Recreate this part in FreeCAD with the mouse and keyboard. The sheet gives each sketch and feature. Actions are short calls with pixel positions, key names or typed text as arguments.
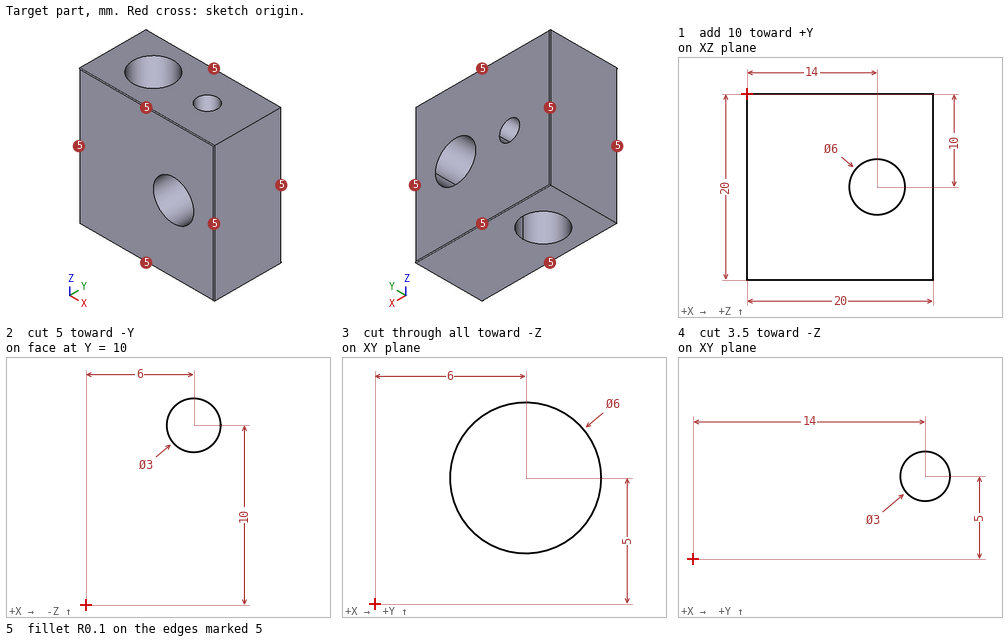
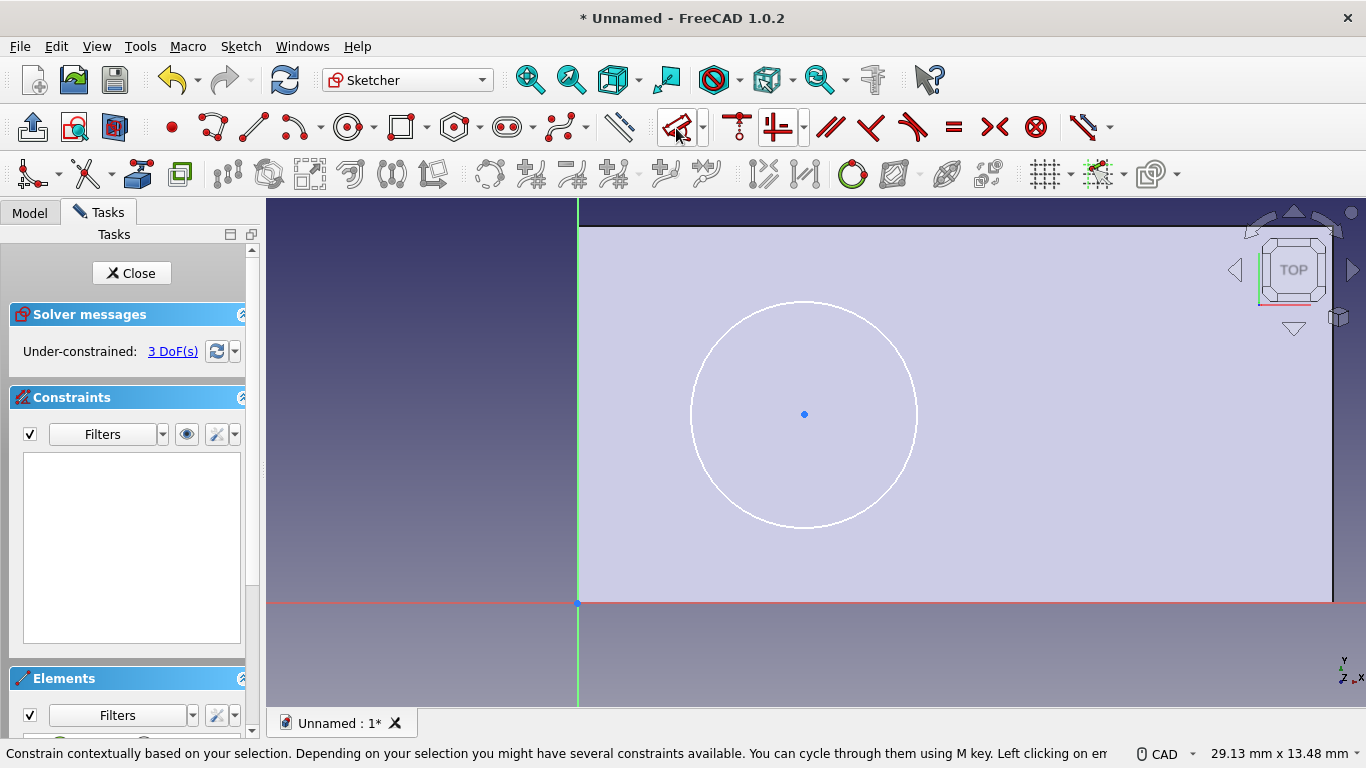
click(884, 335)
click(907, 312)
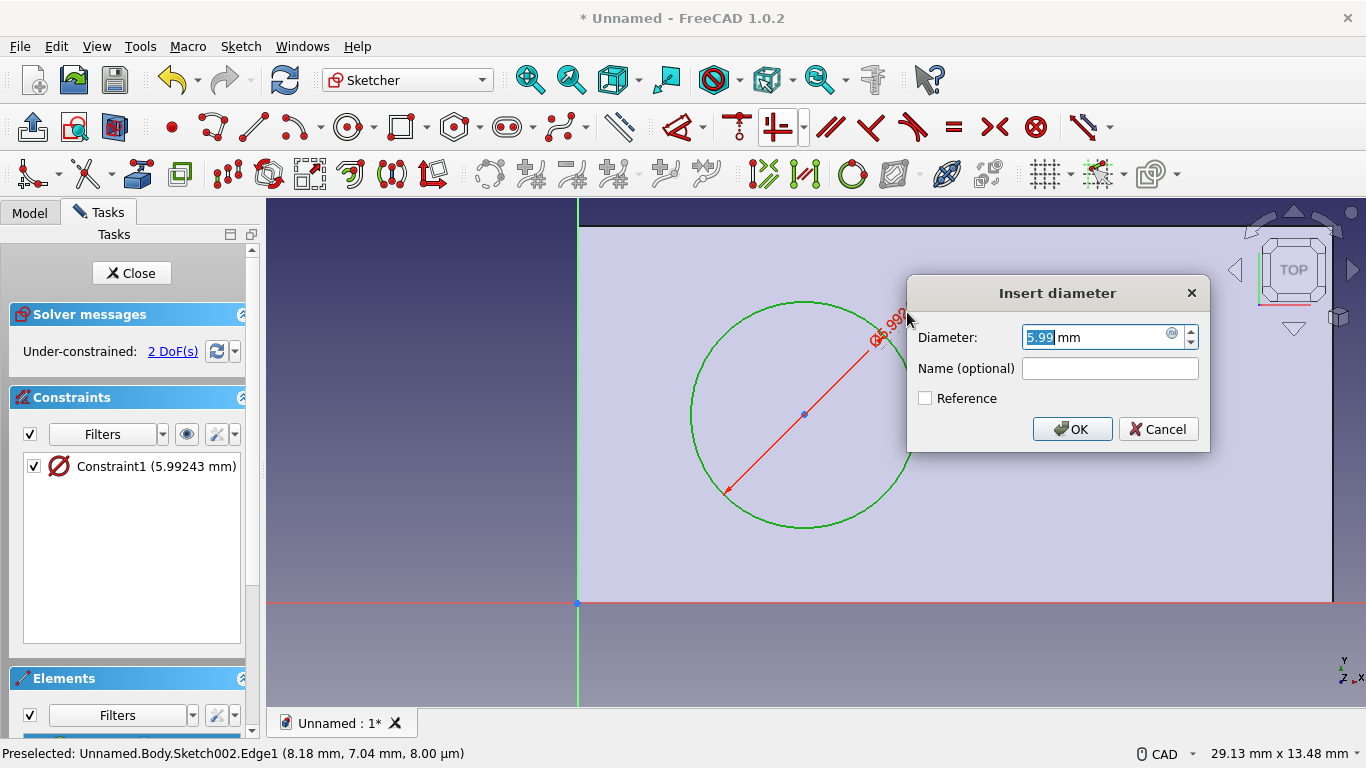
text(6)
key(Return)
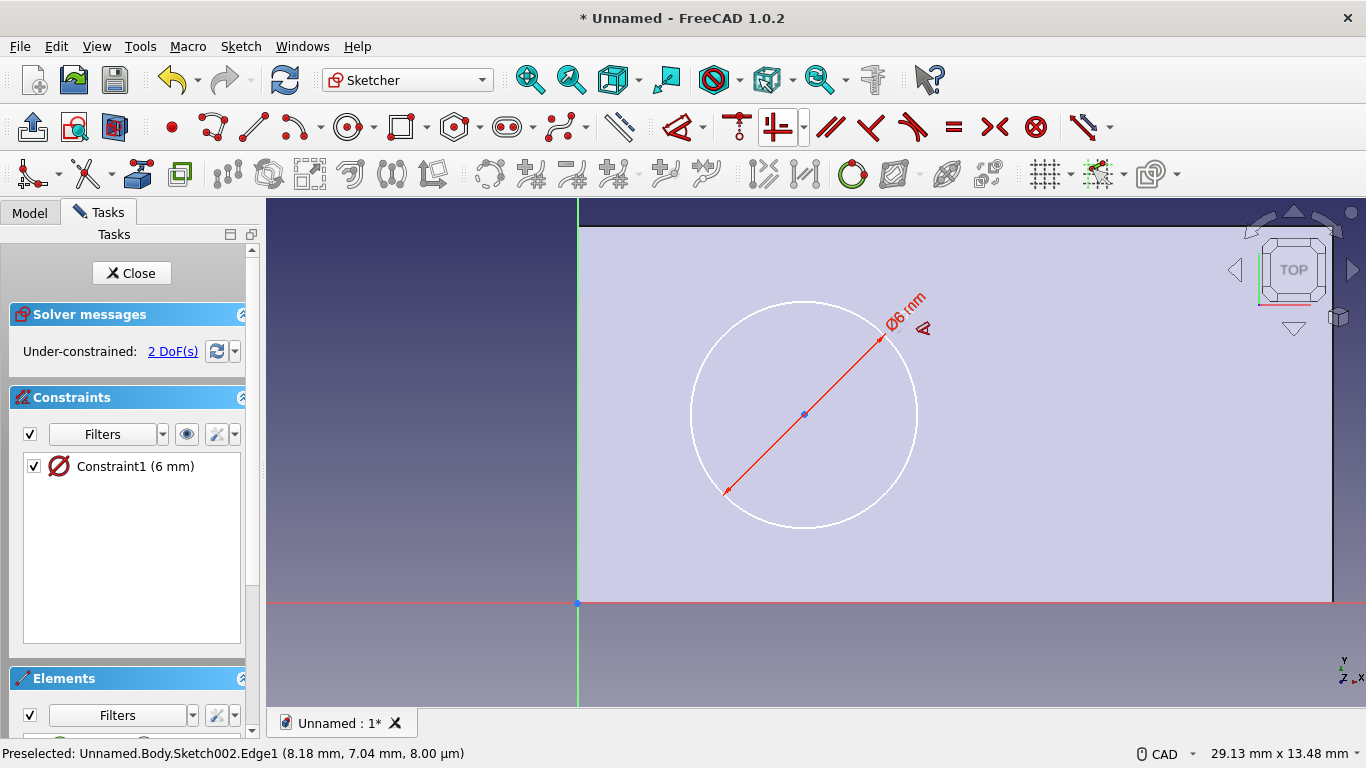
click(804, 415)
click(691, 637)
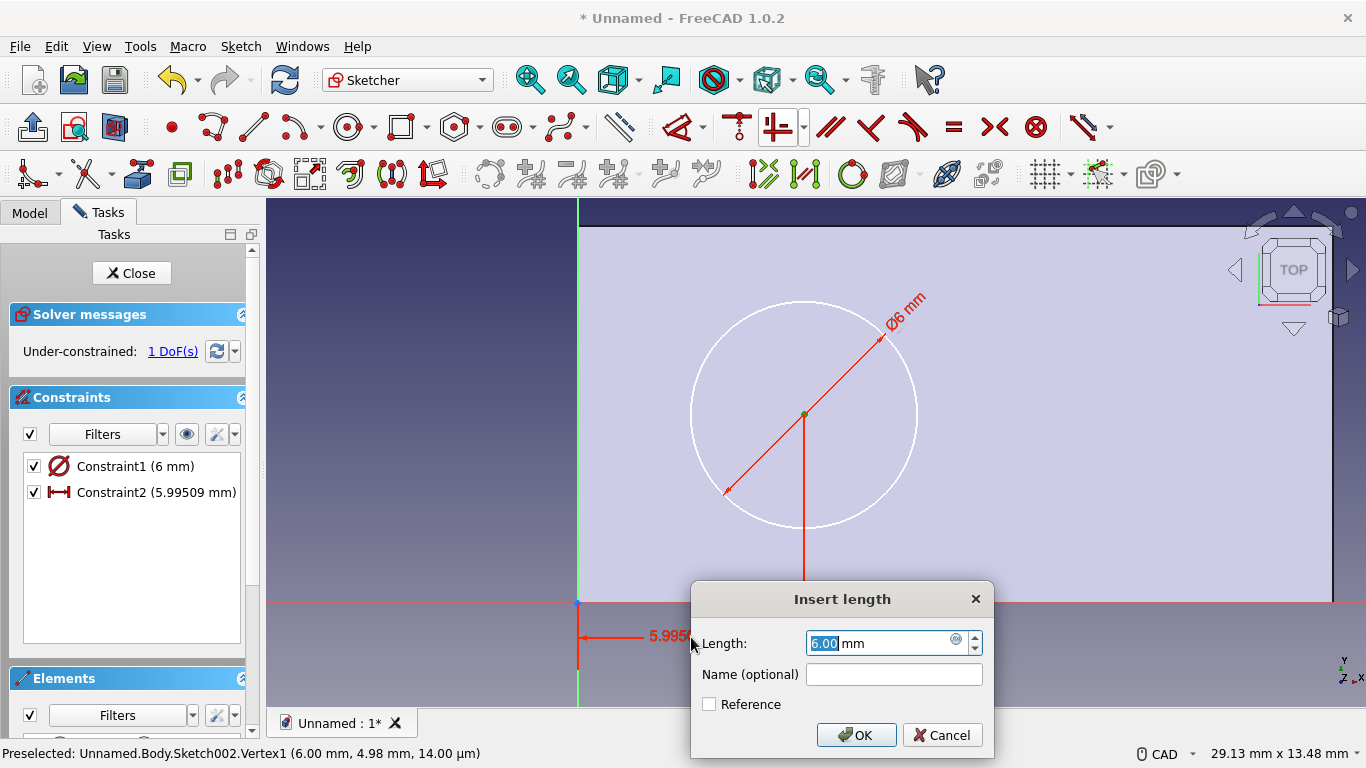
text(6)
key(Return)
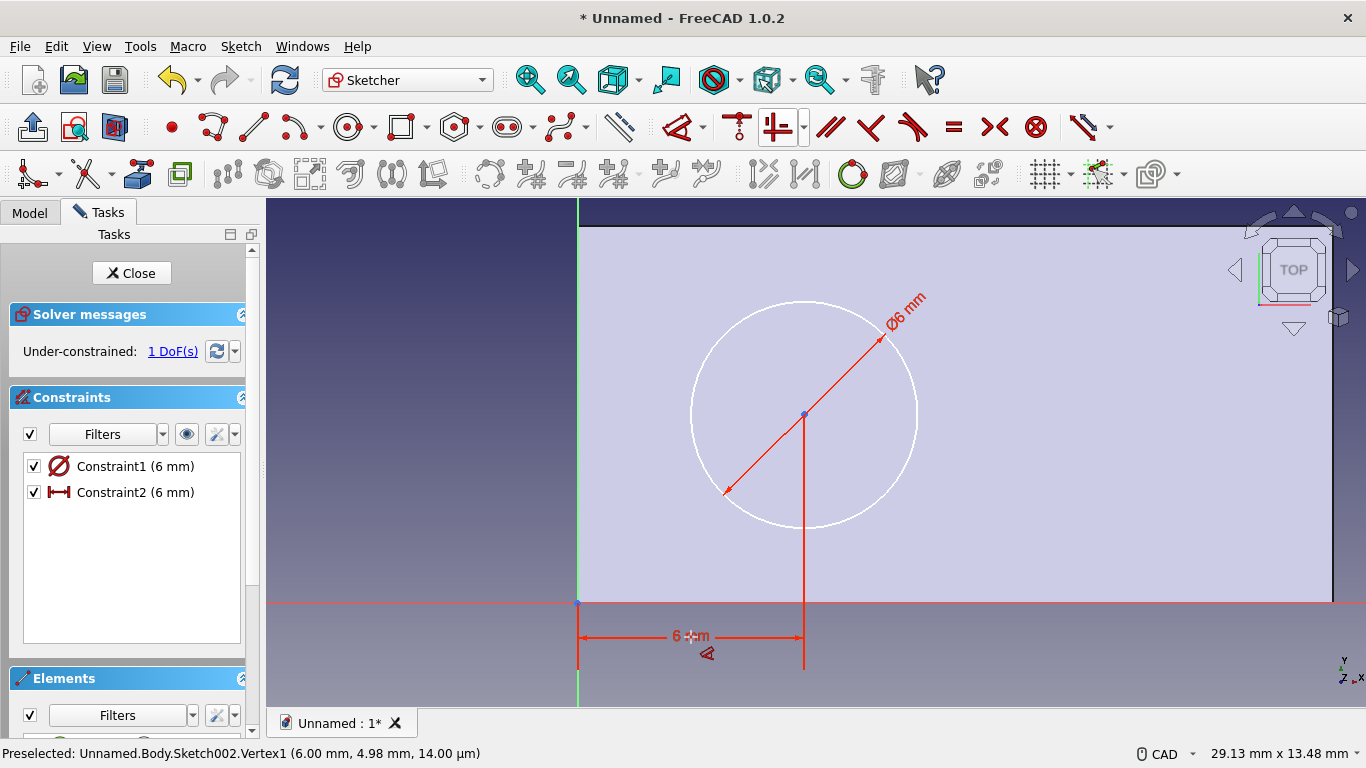
click(804, 415)
click(544, 509)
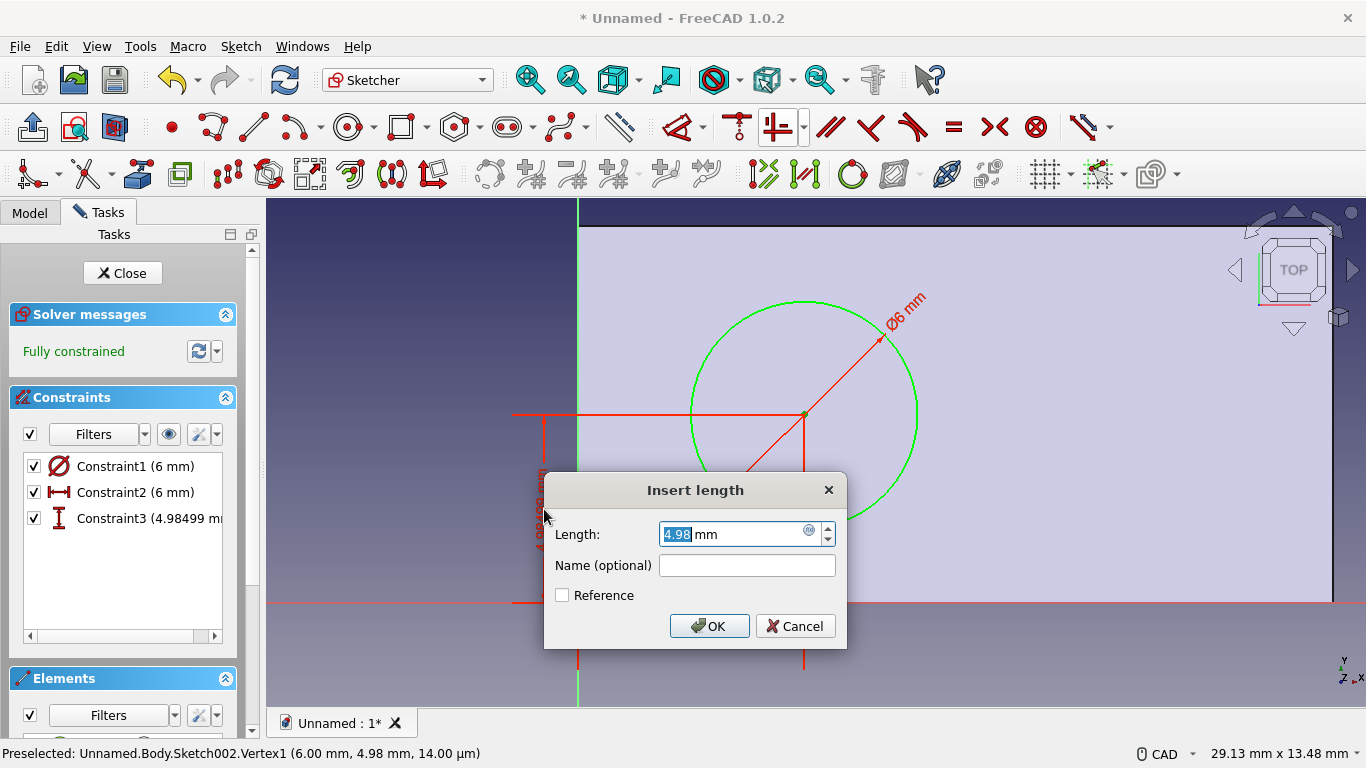
text(5)
key(Return)
key(Escape)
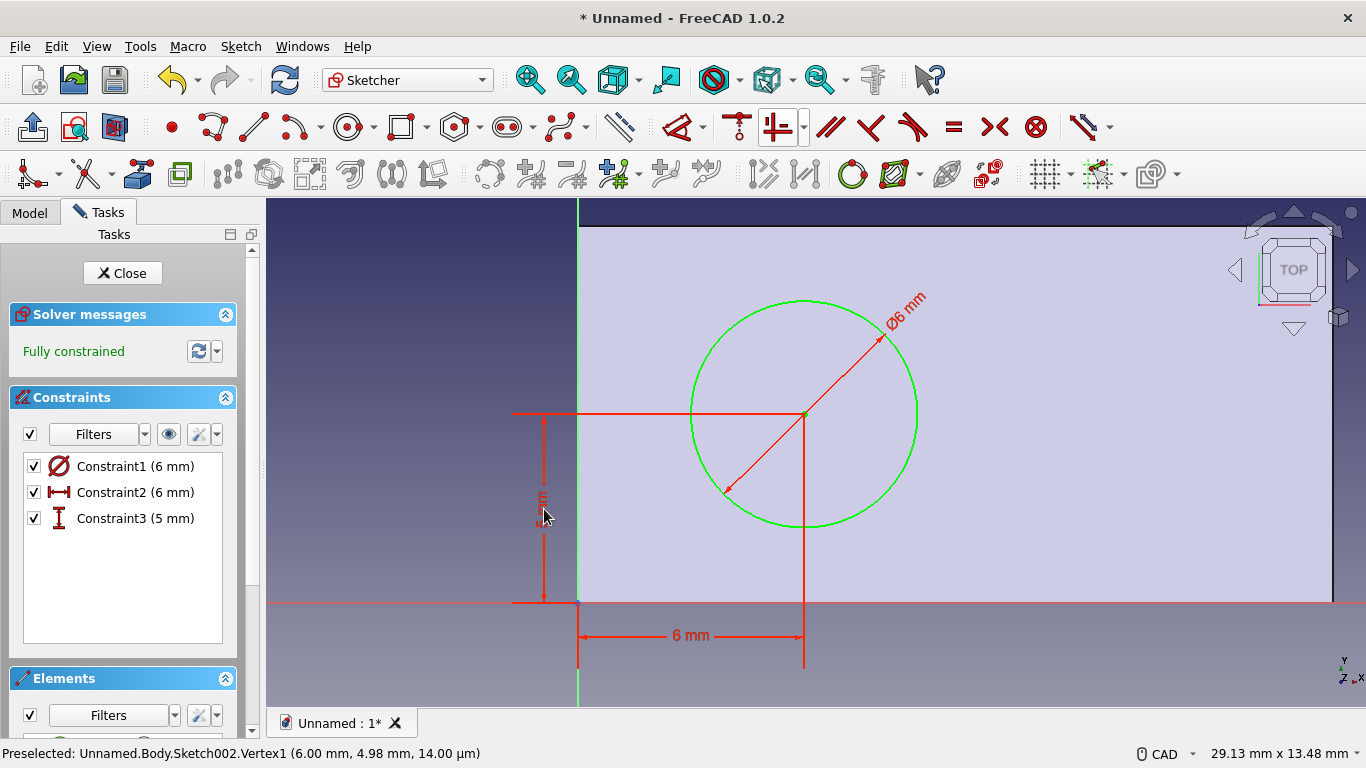
click(123, 273)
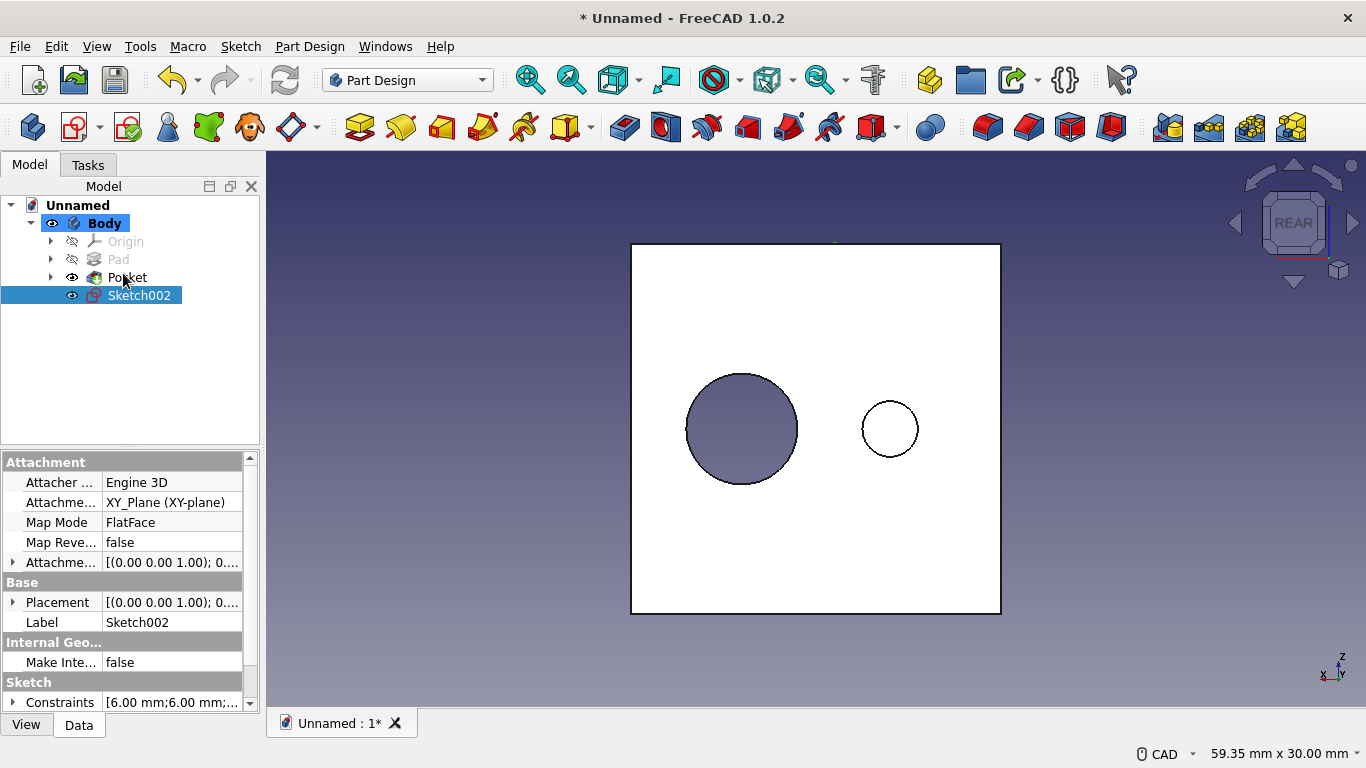
click(625, 128)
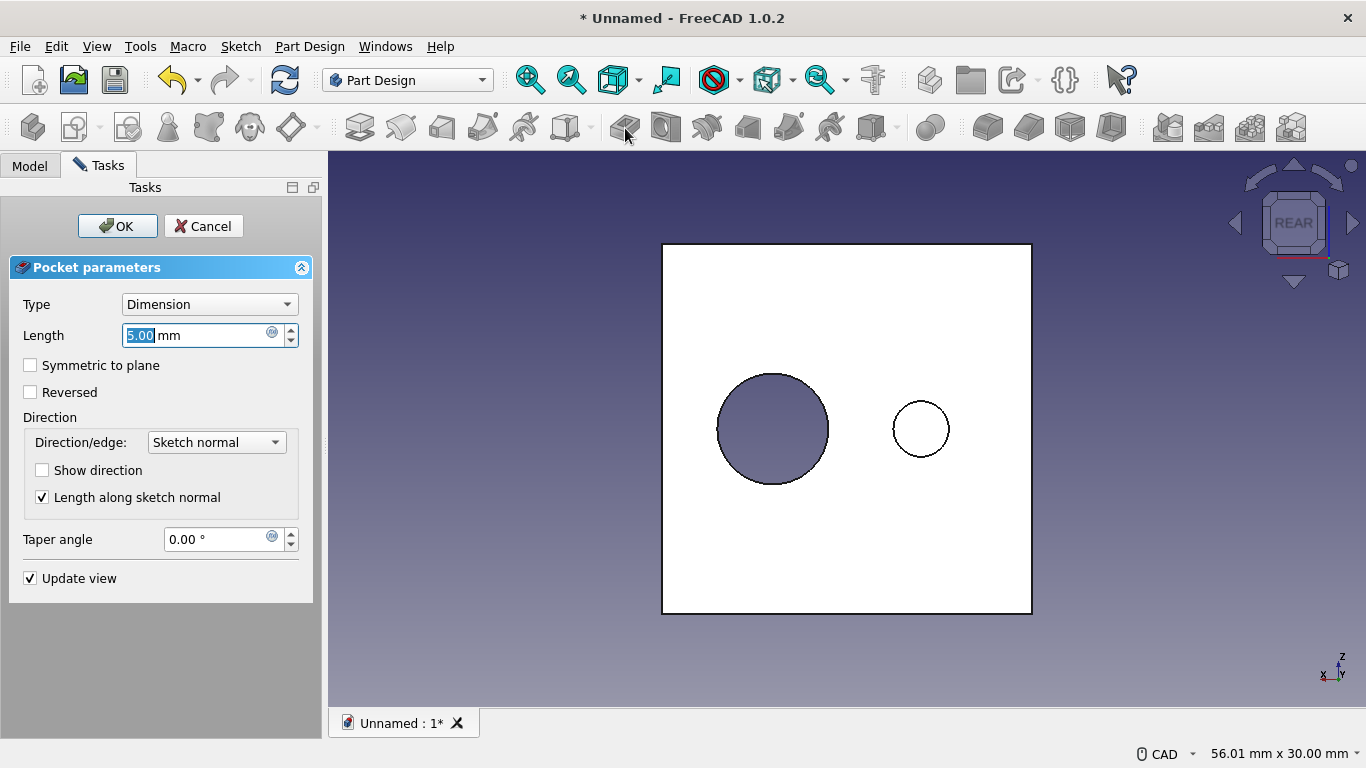
click(210, 304)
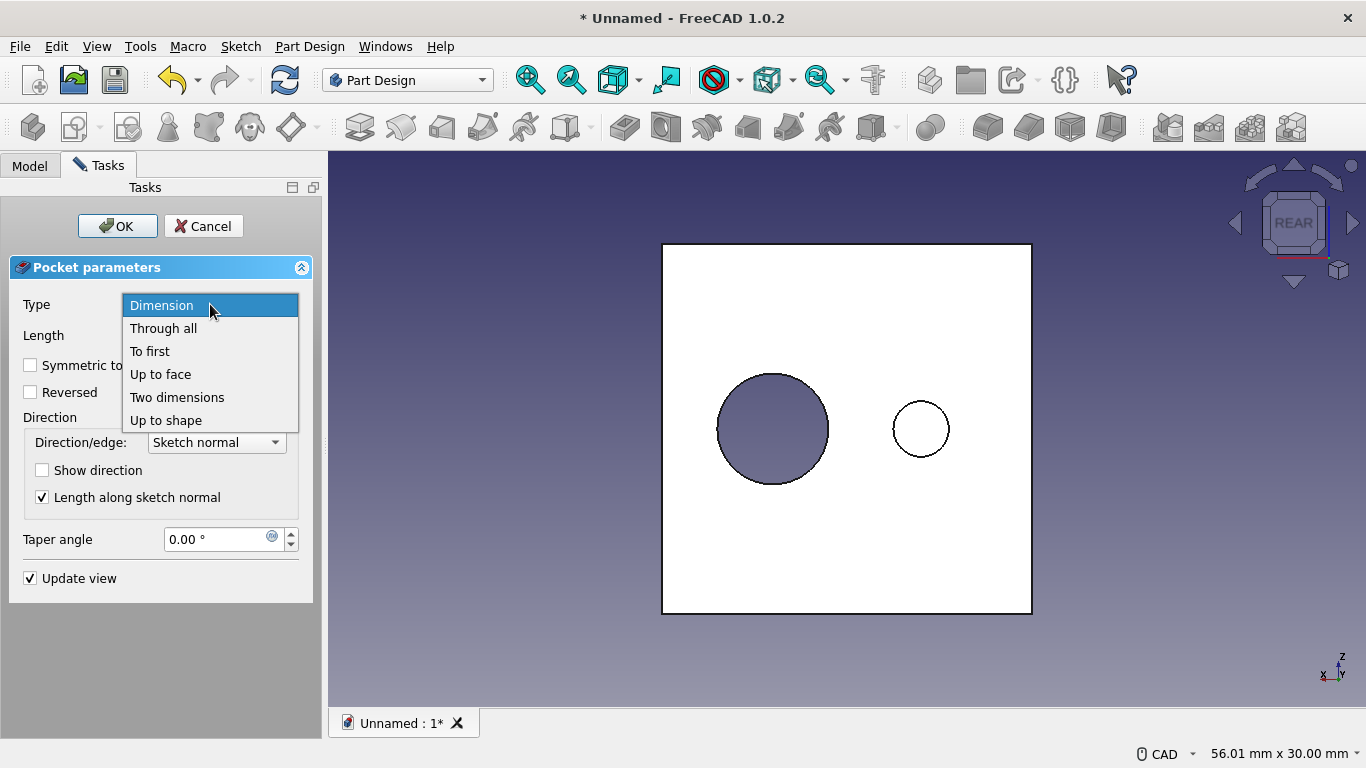
click(208, 328)